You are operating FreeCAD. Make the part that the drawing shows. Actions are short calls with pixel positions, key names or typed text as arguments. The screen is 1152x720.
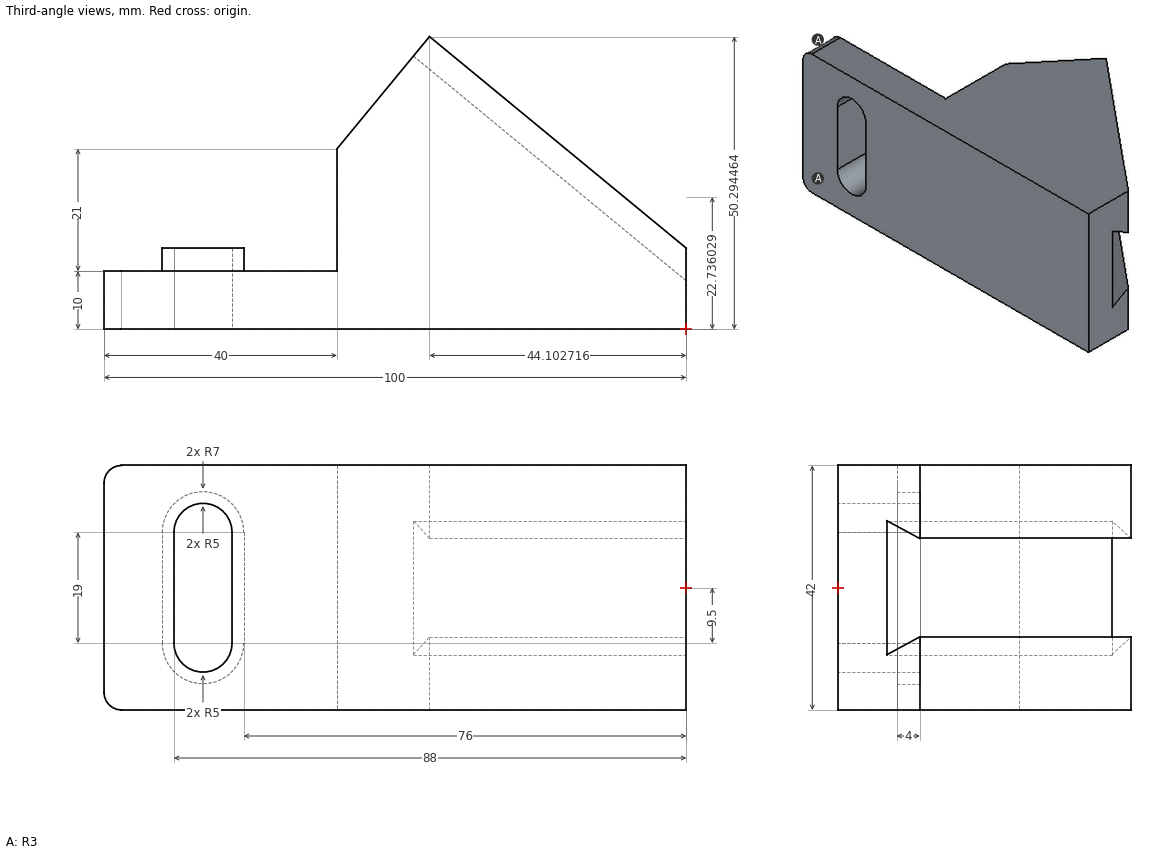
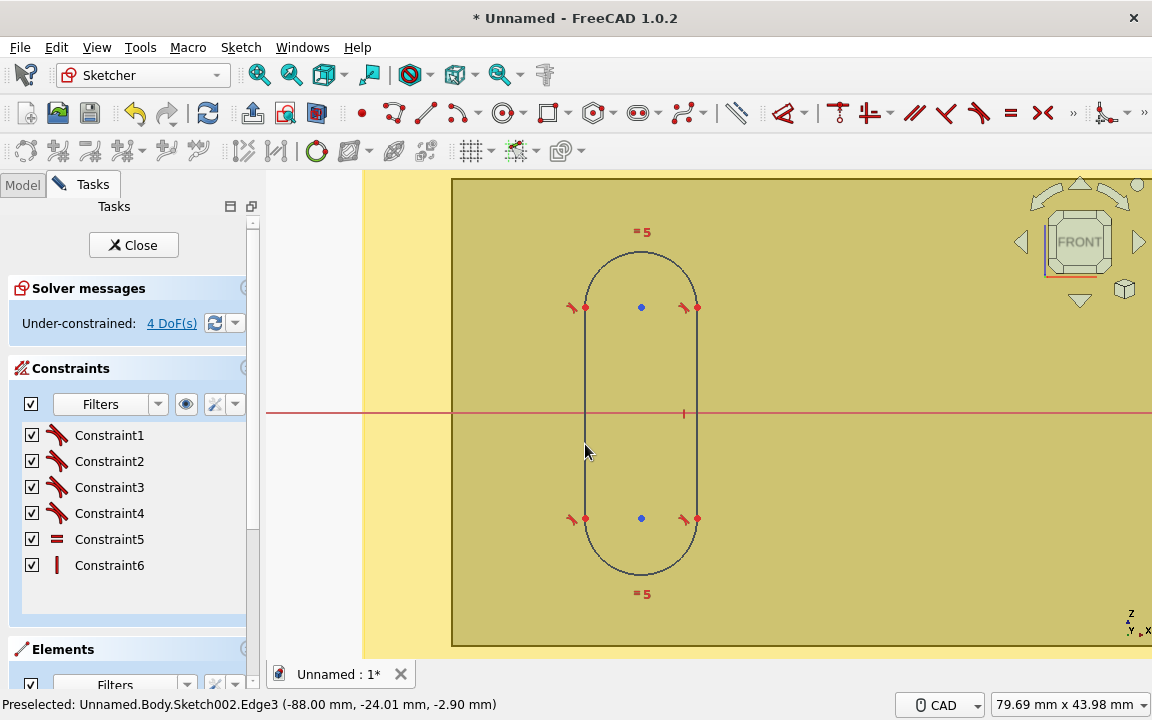
key(d)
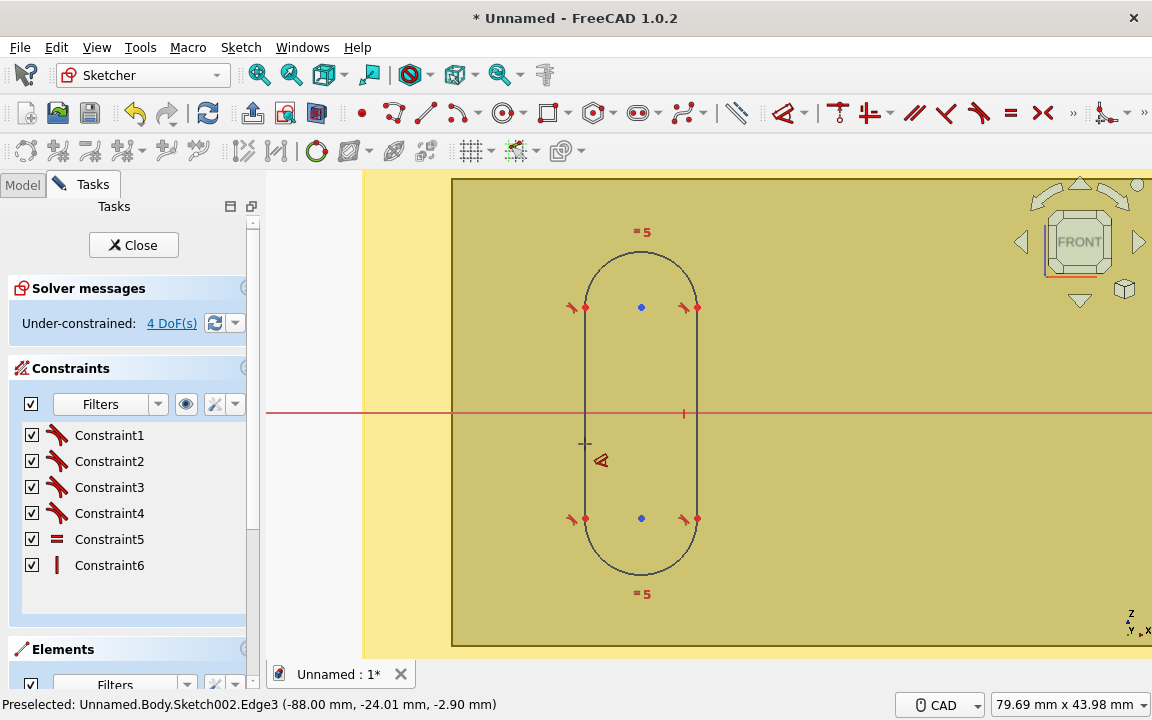
click(608, 564)
click(589, 590)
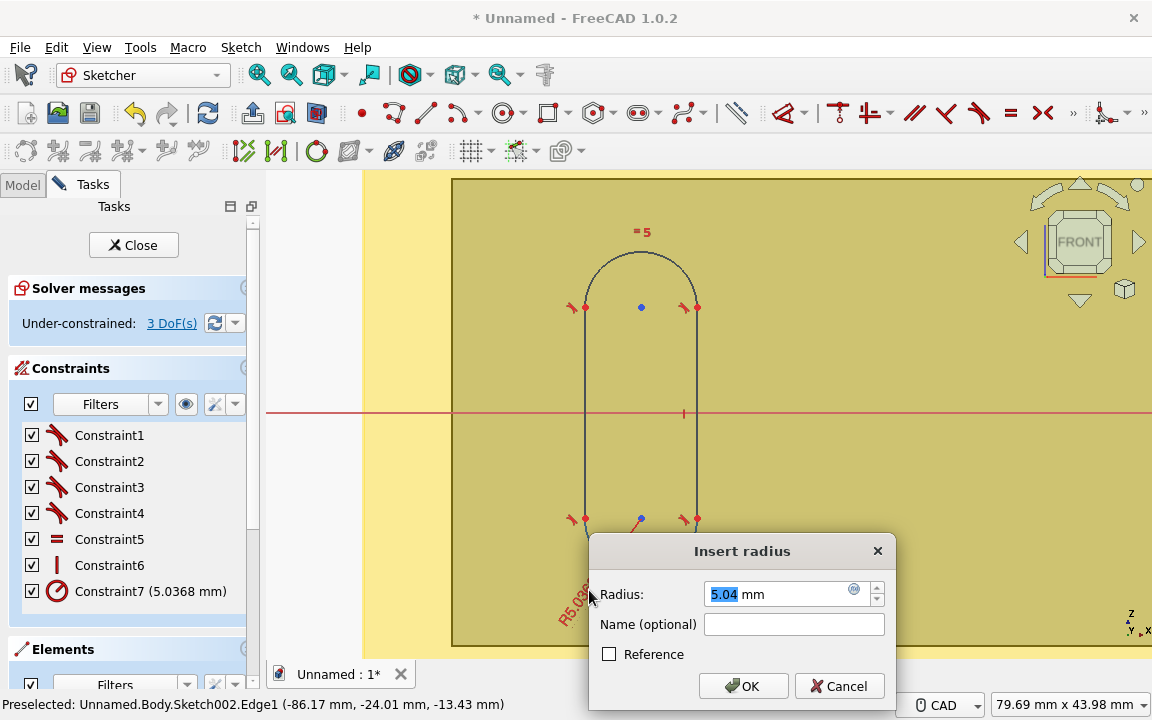
text(5)
key(Return)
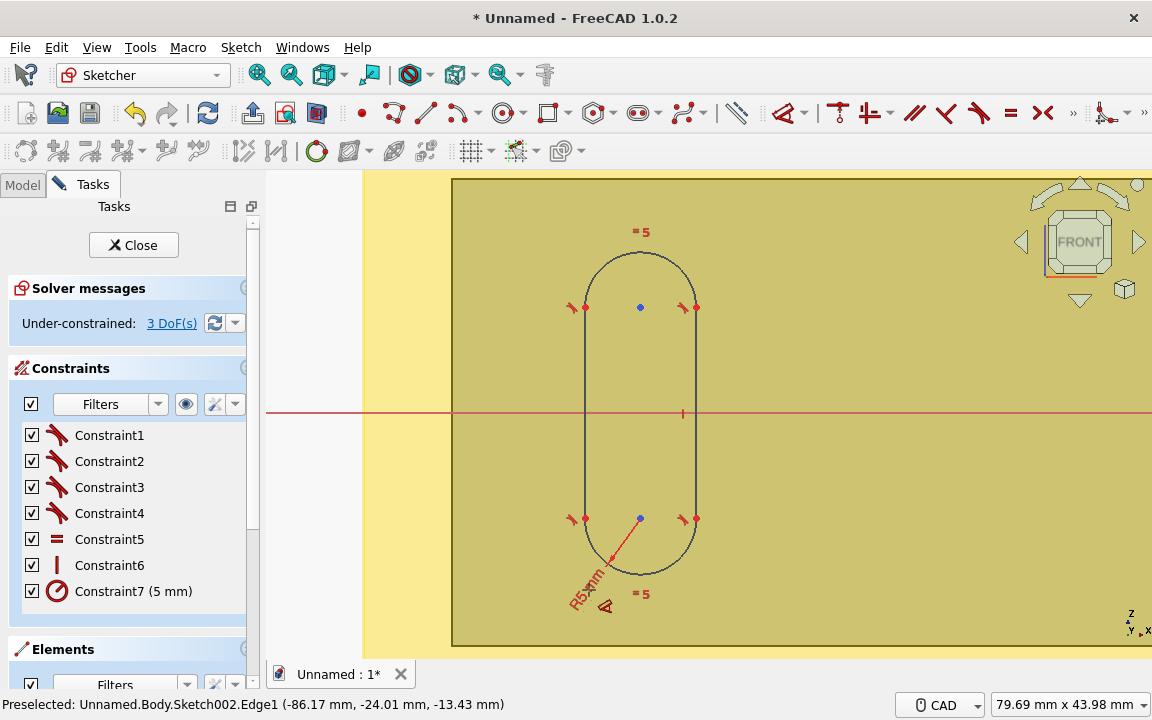
click(585, 456)
click(551, 365)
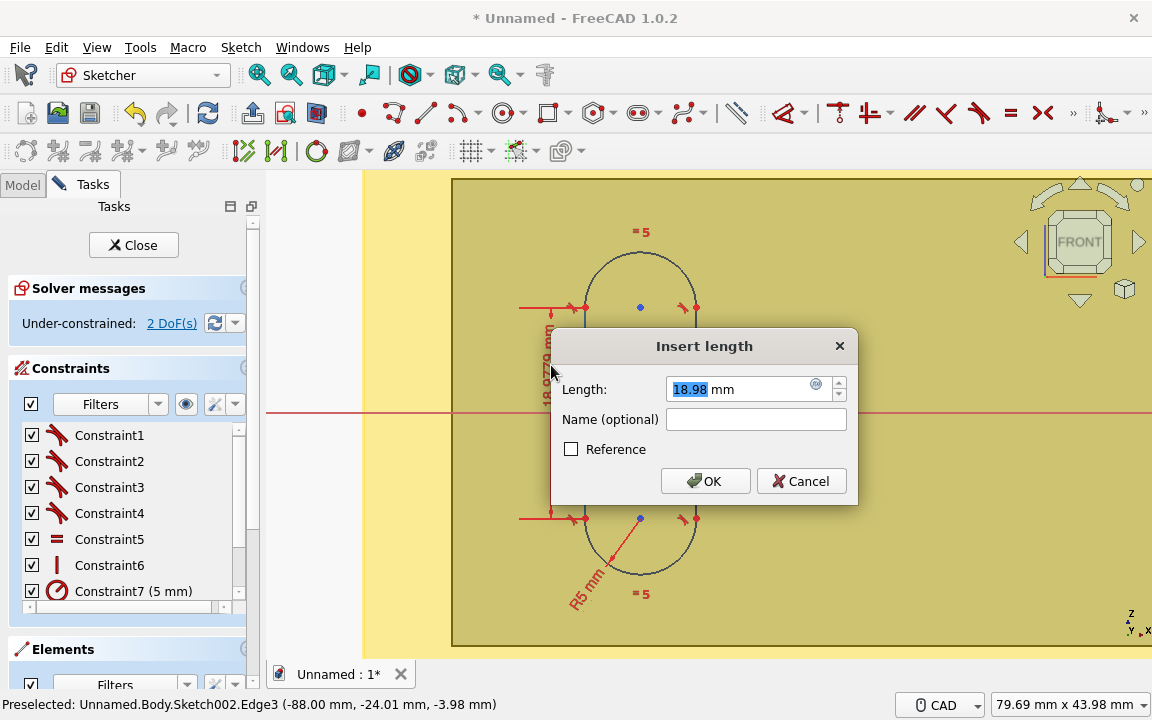
text(19)
key(Return)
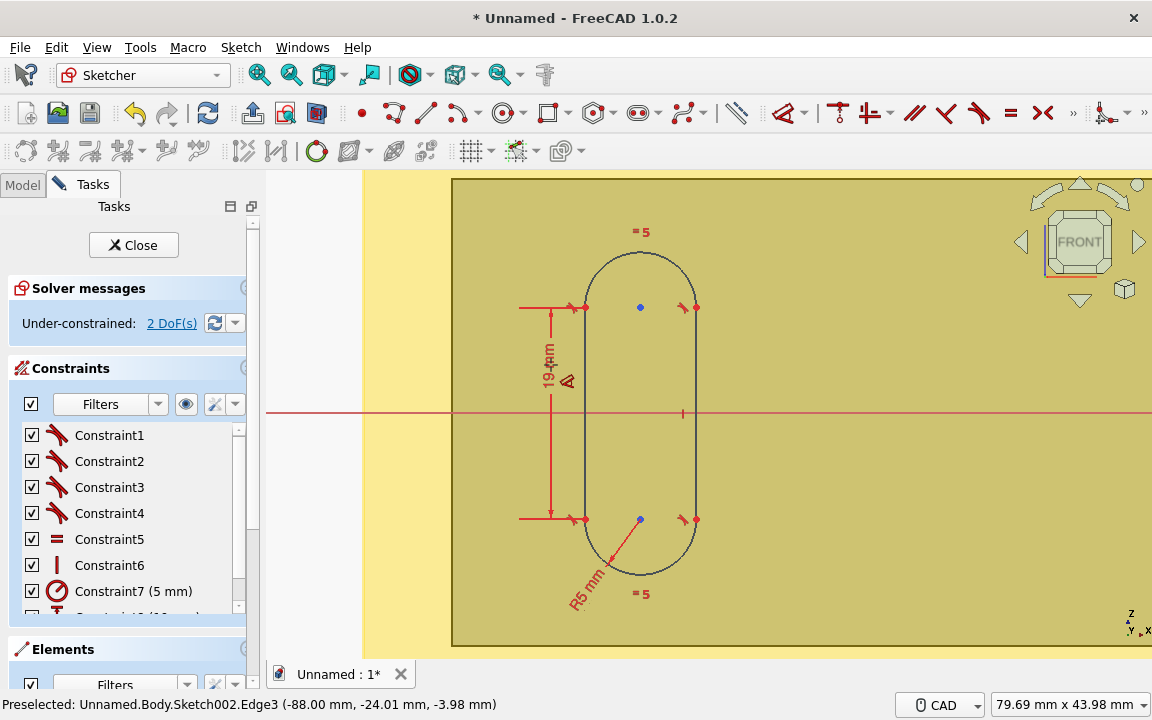
click(585, 519)
click(786, 553)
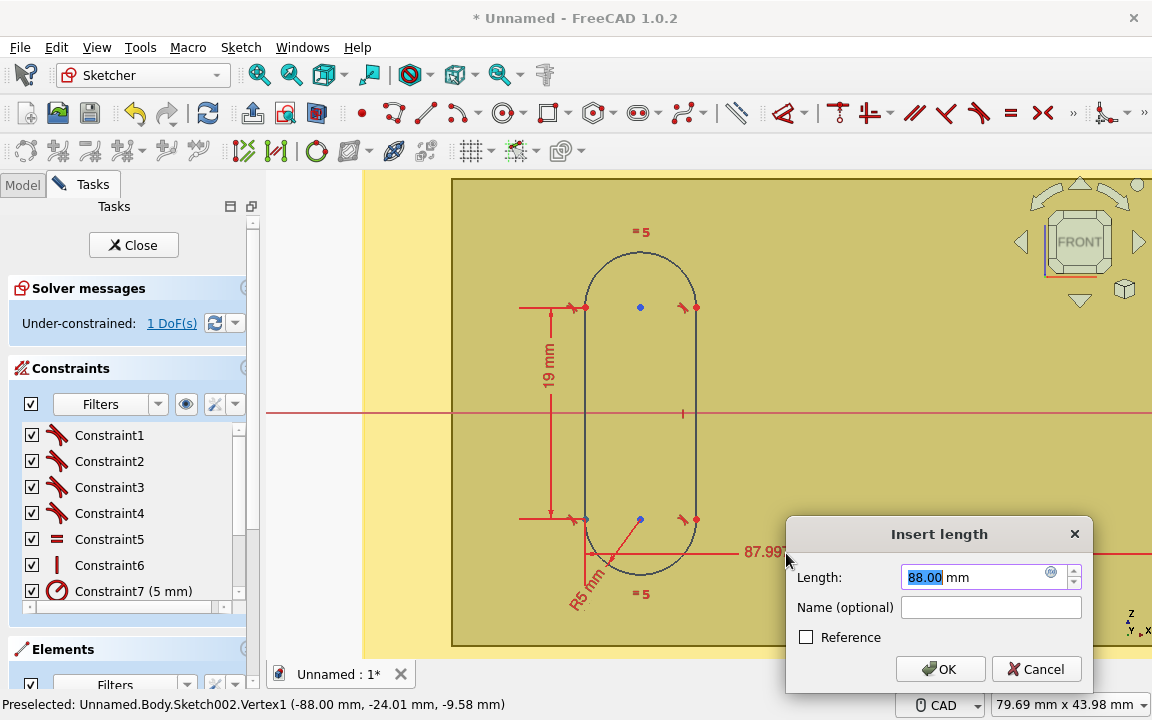
text(88)
key(Return)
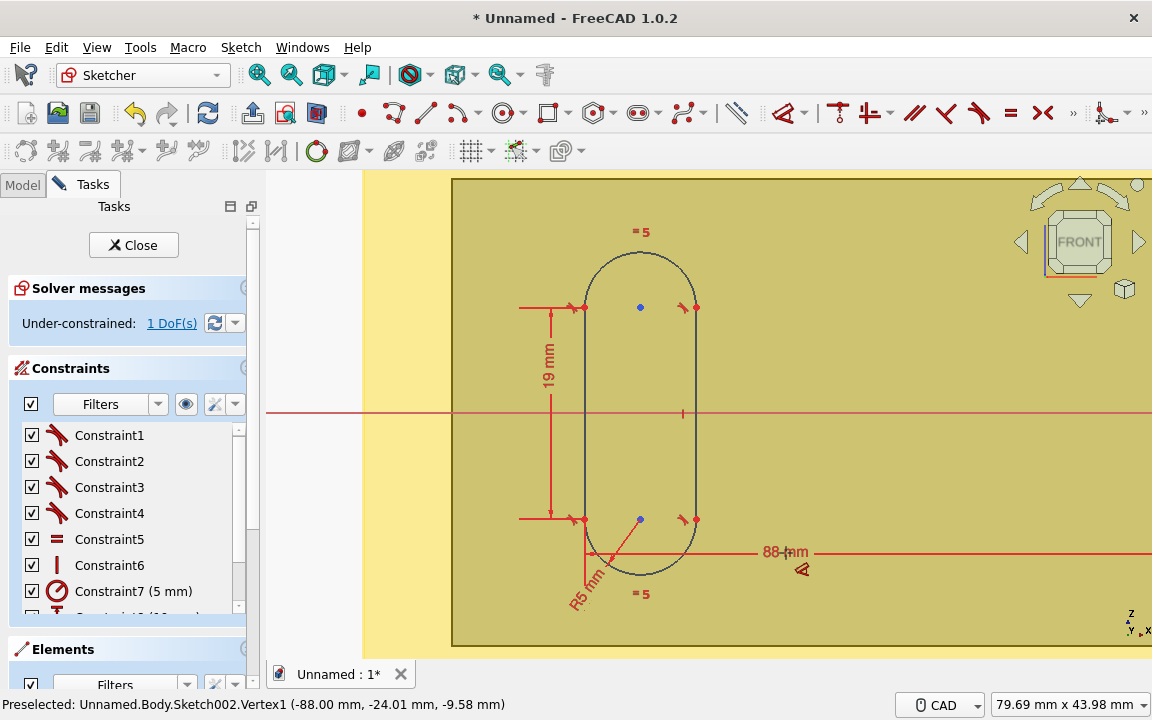
click(585, 519)
click(551, 466)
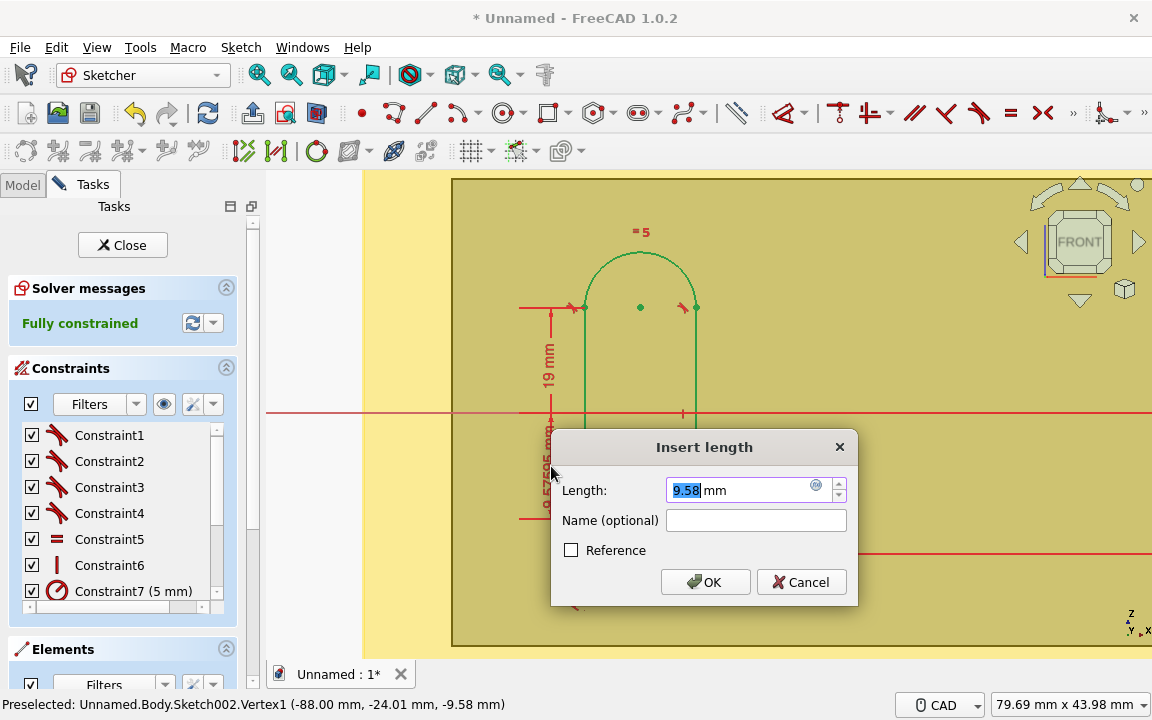
text(9.5)
key(Return)
key(Escape)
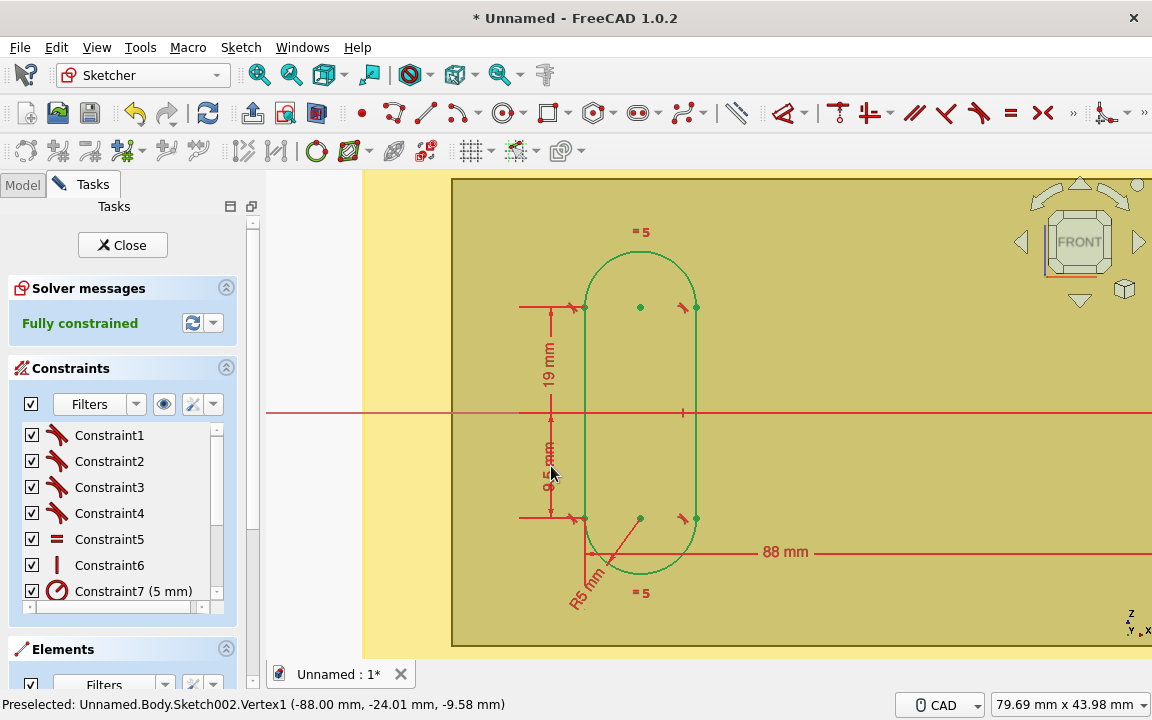
click(123, 245)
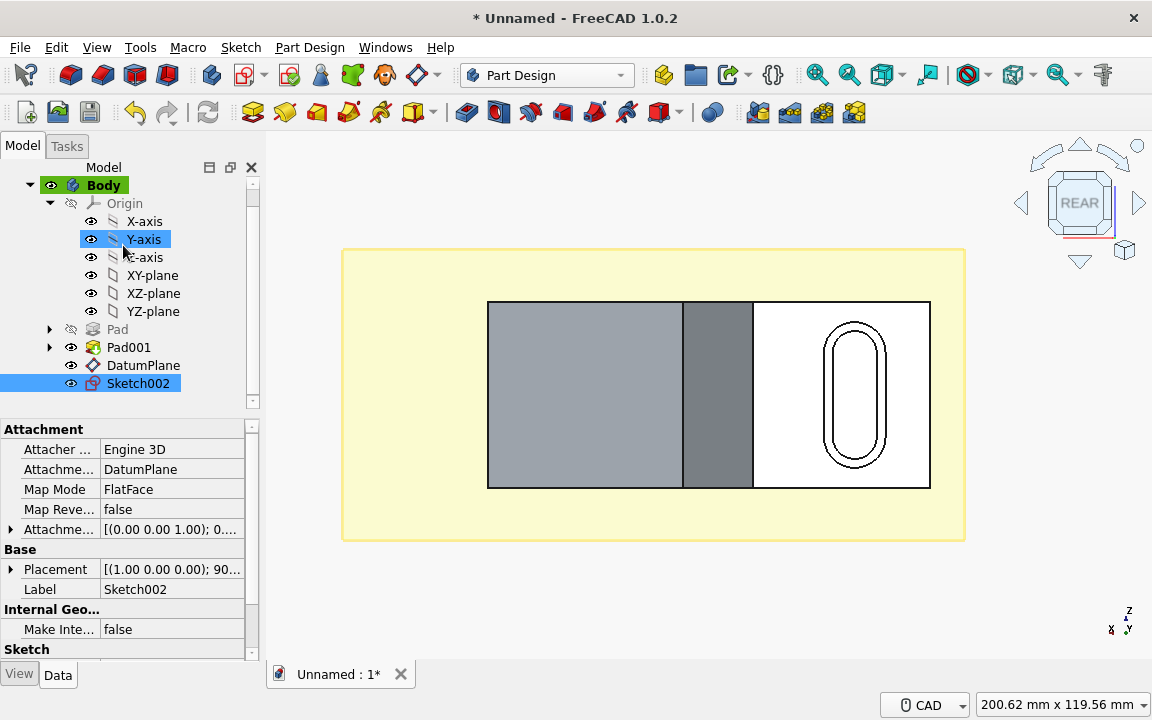
click(468, 112)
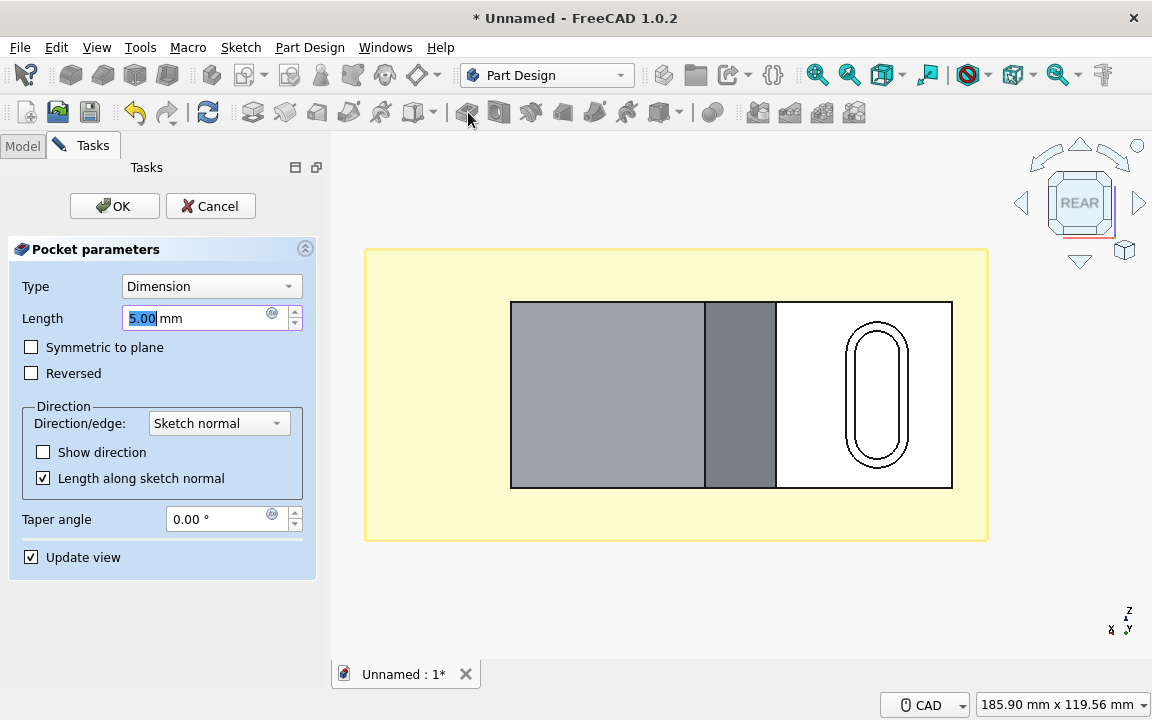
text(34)
key(Tab)